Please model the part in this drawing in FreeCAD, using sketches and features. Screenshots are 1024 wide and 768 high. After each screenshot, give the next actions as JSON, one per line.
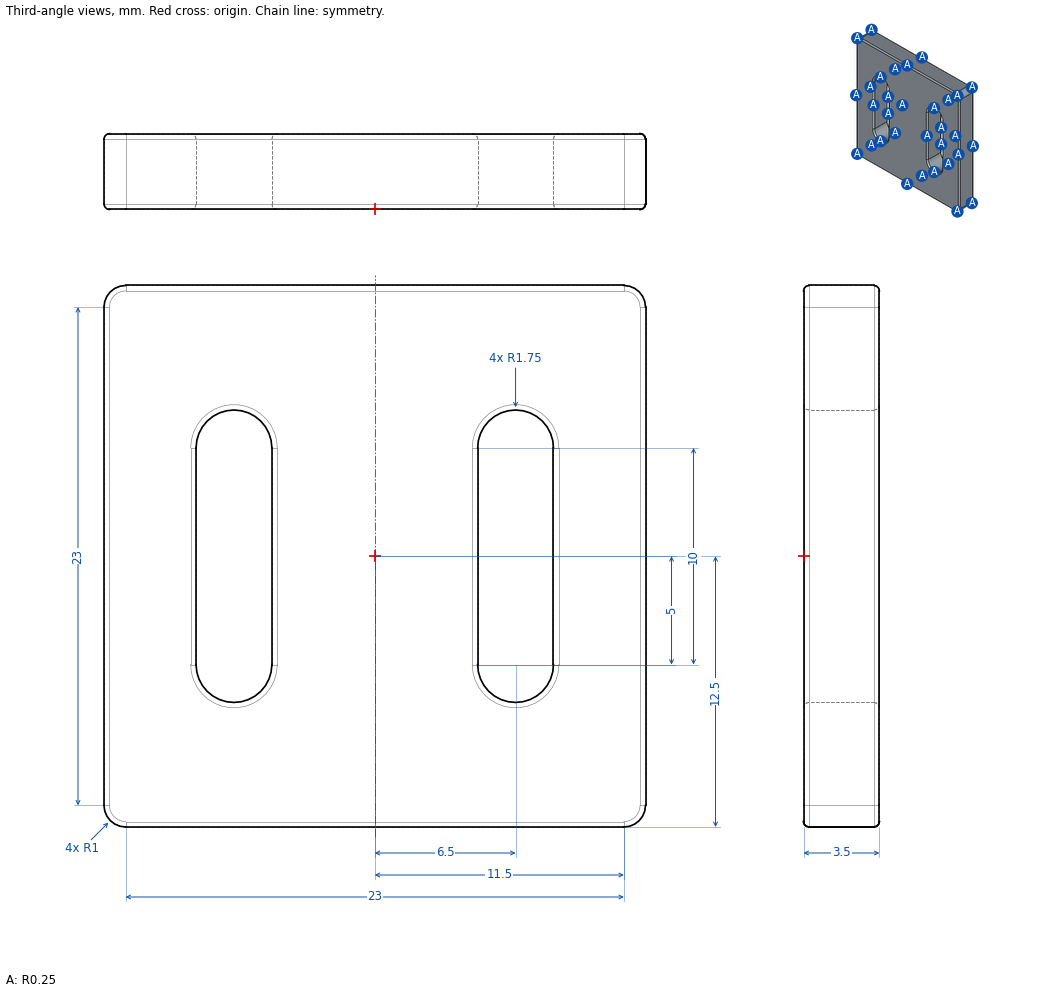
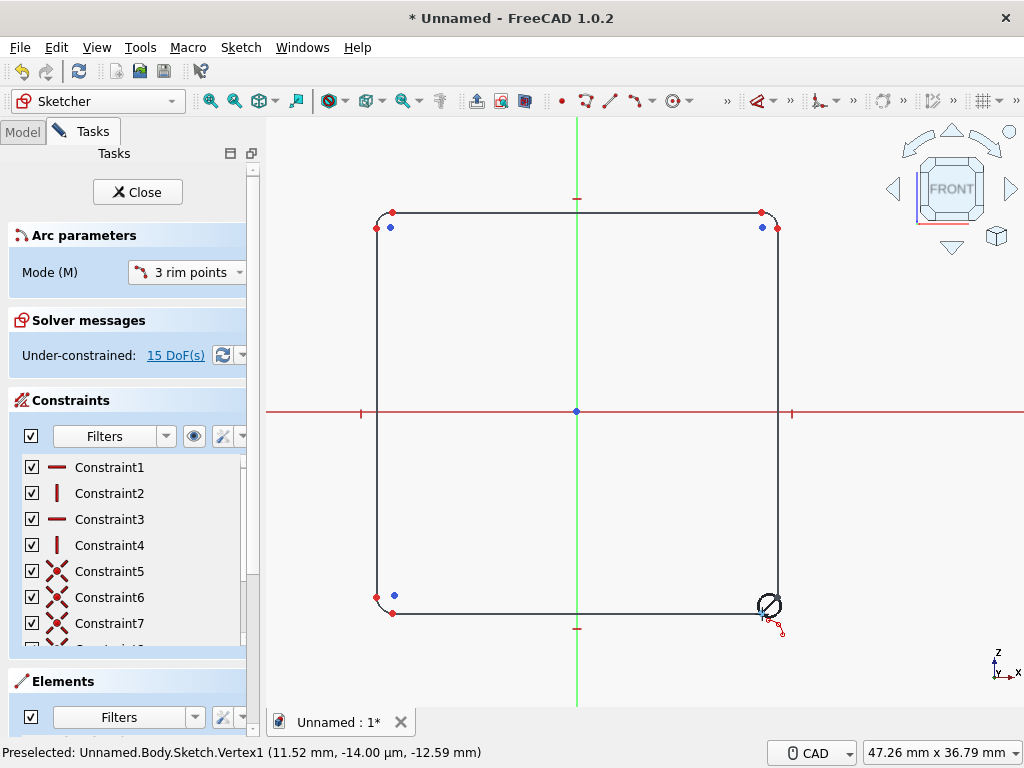
{"action": "scroll", "coordinate": [773, 608], "scroll_direction": "up", "scroll_amount": 7}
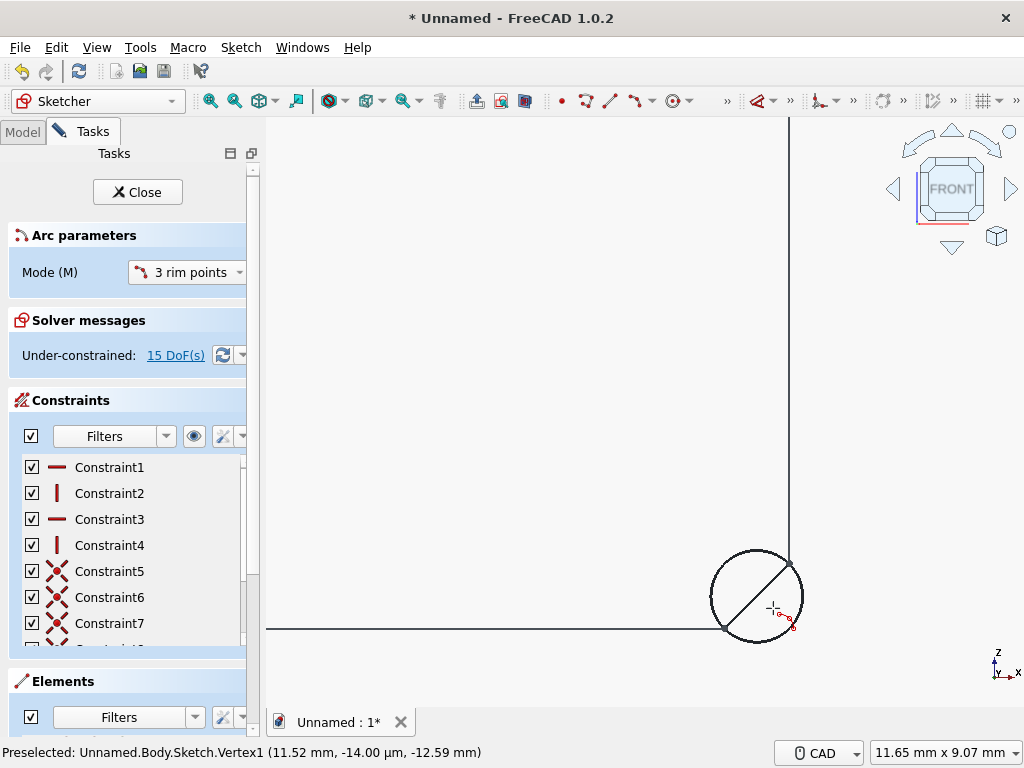
{"action": "left_click", "coordinate": [769, 604]}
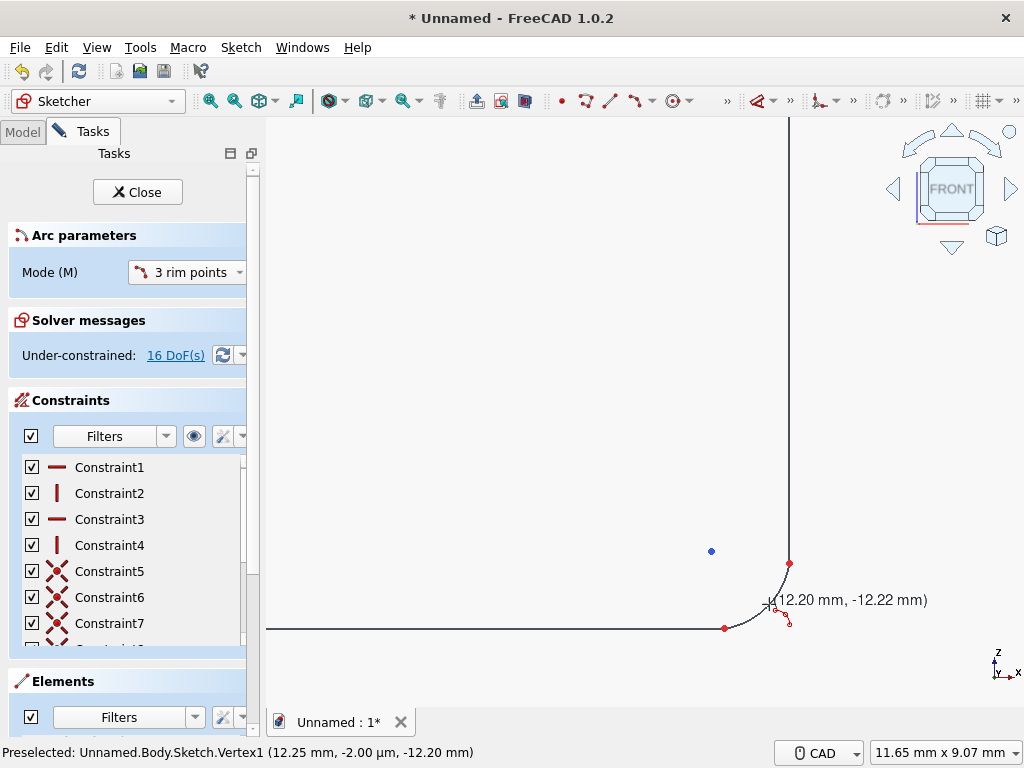
{"action": "key", "text": "g s"}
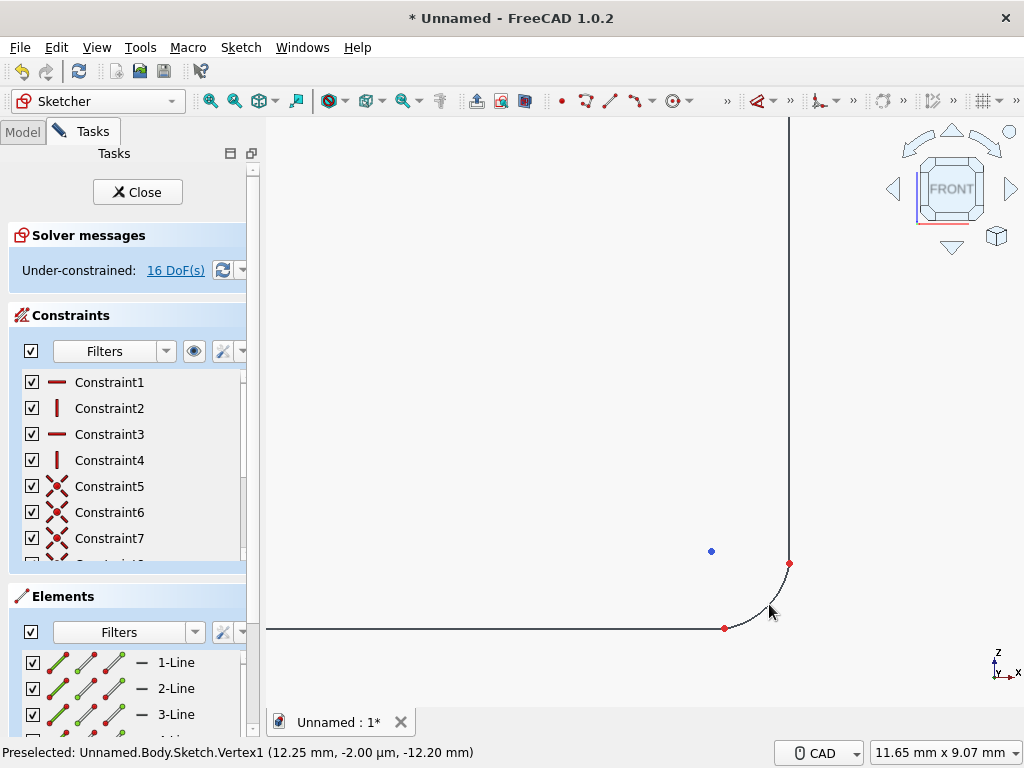
{"action": "scroll", "coordinate": [773, 609], "scroll_direction": "down", "scroll_amount": 7}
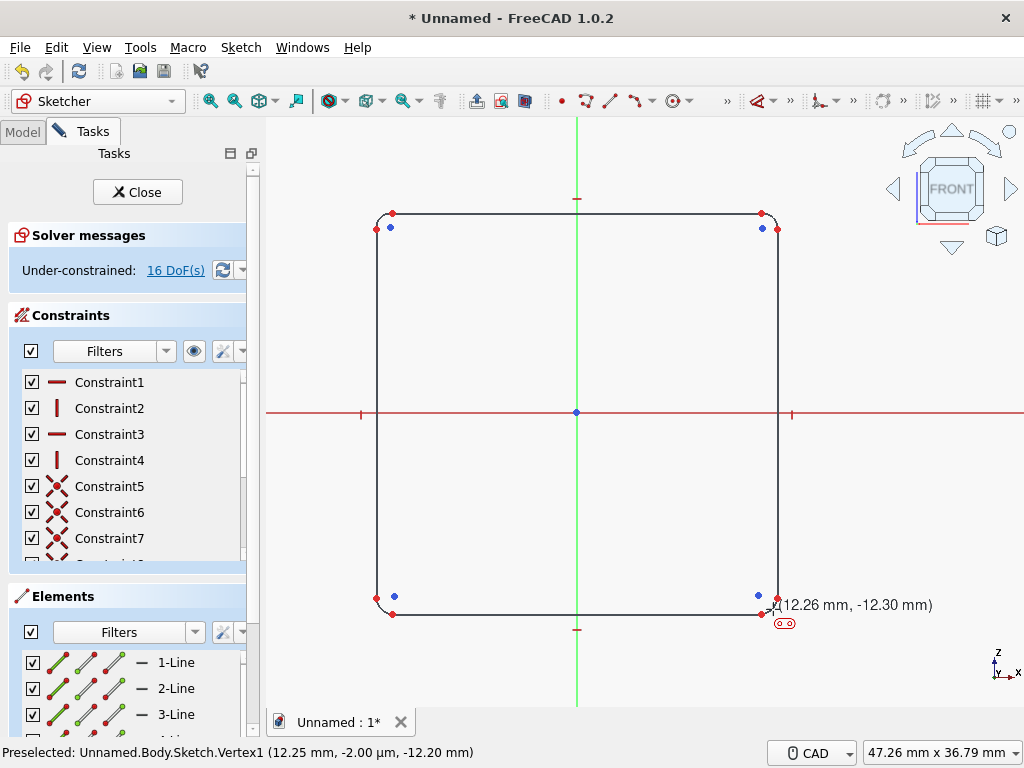
{"action": "left_click", "coordinate": [681, 493]}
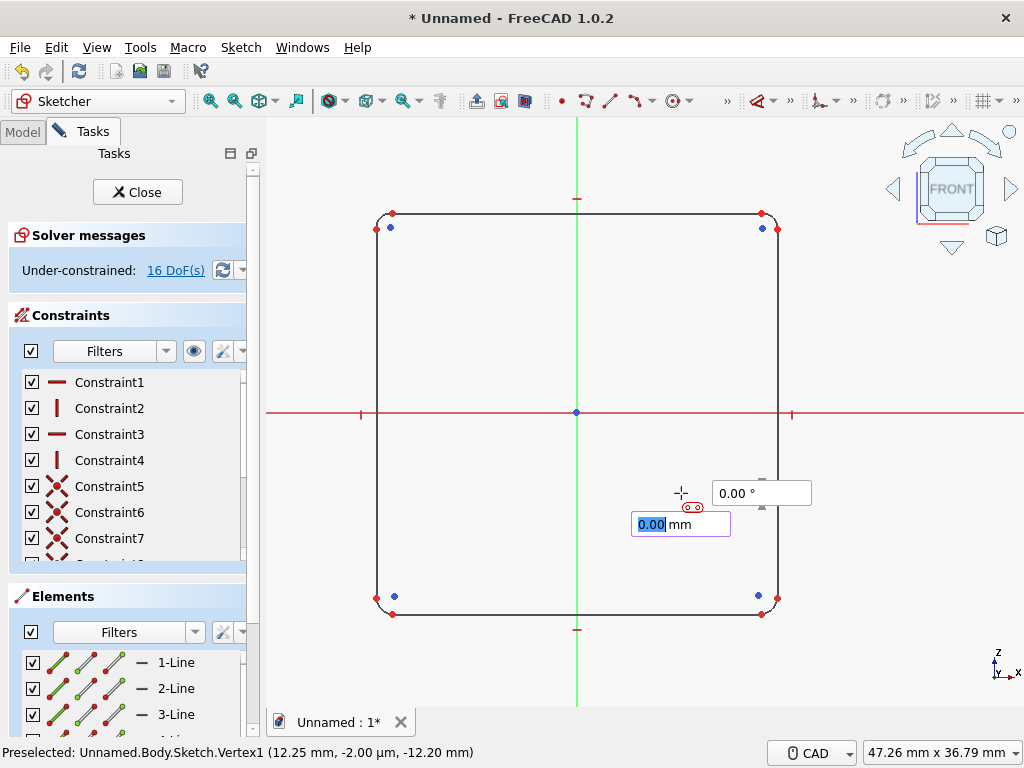
{"action": "left_click", "coordinate": [681, 332]}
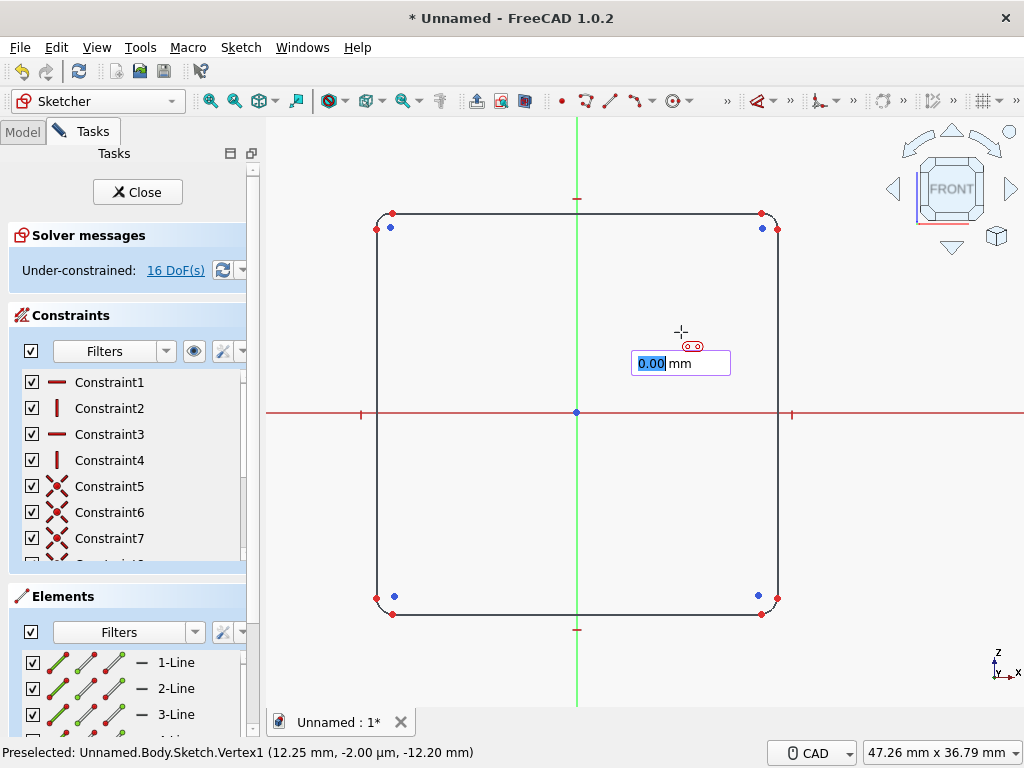
{"action": "left_click", "coordinate": [653, 389]}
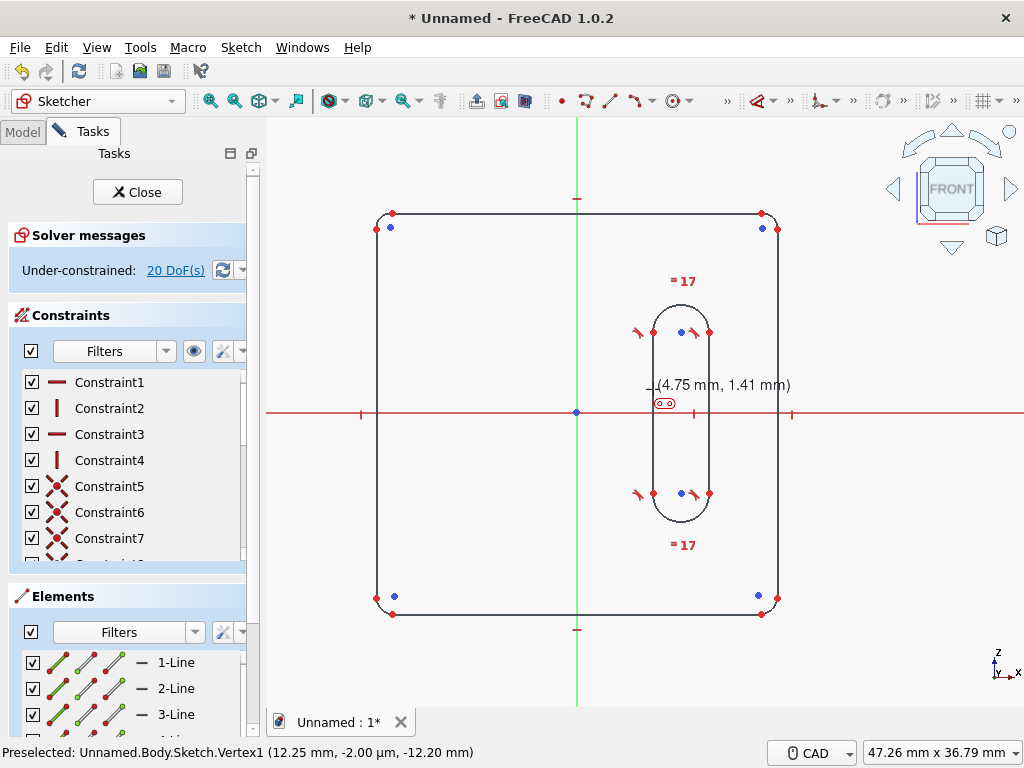
{"action": "left_click", "coordinate": [473, 493]}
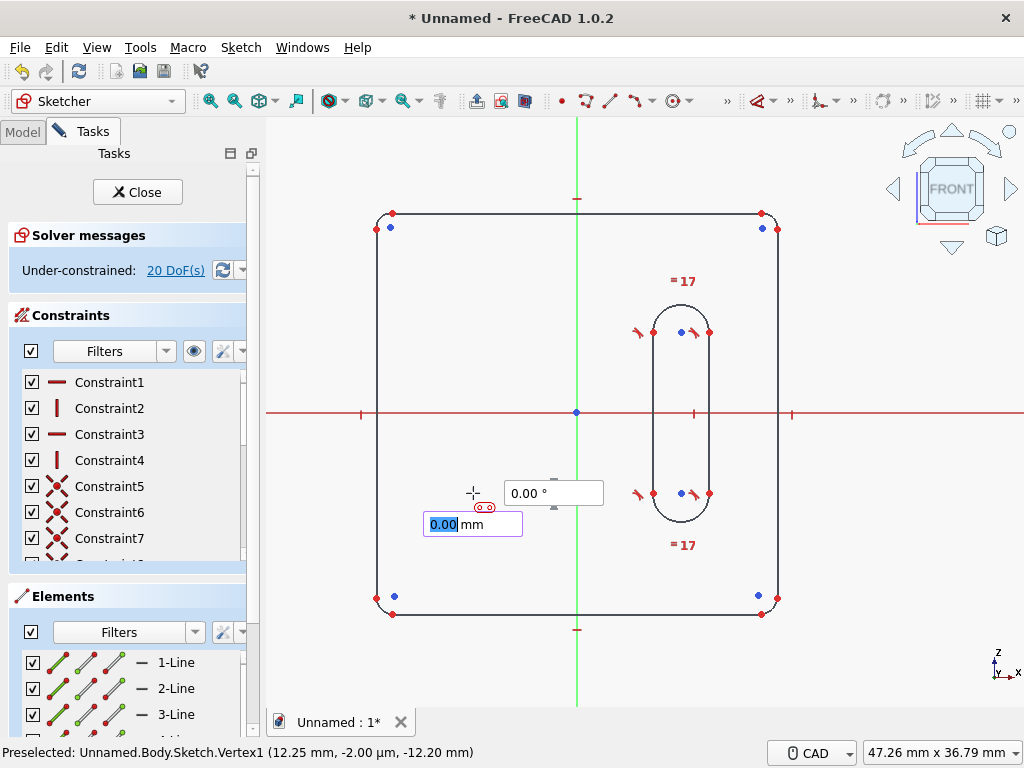
{"action": "left_click", "coordinate": [473, 332]}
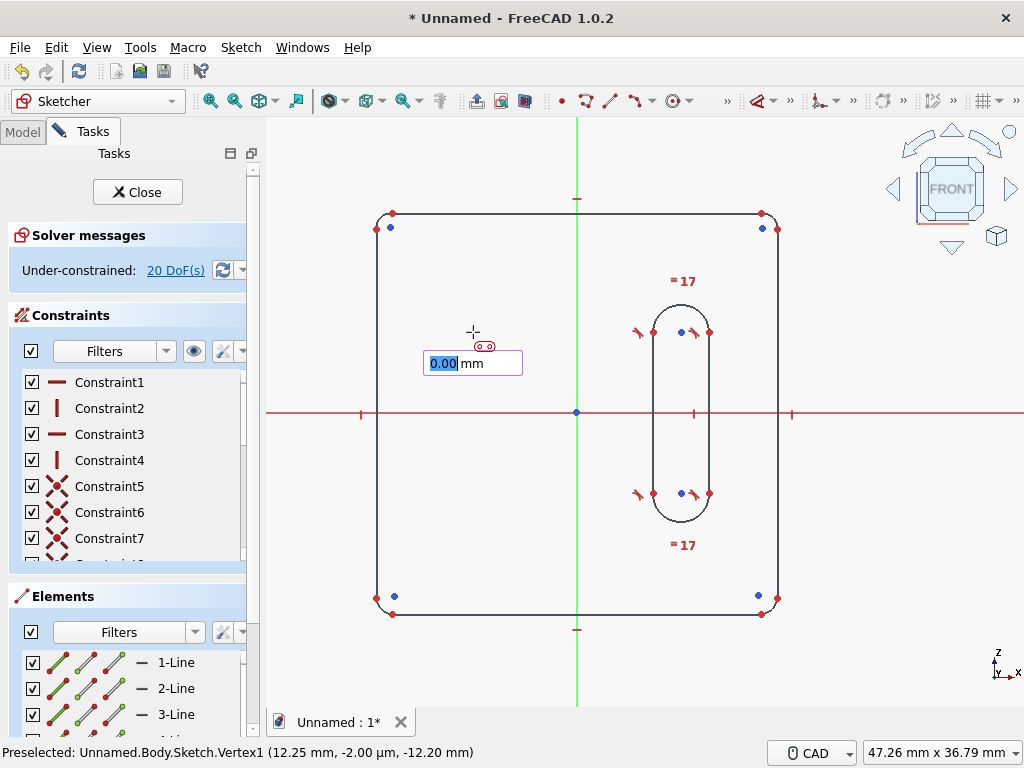
{"action": "left_click", "coordinate": [445, 389]}
{"action": "key", "text": "Escape"}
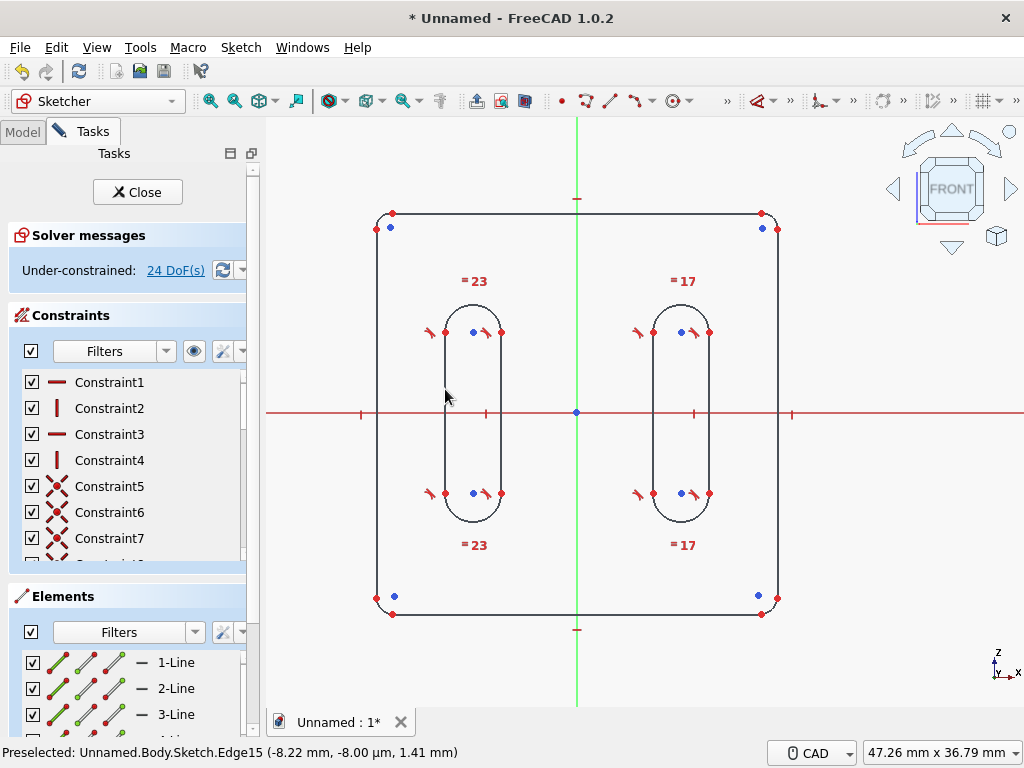
{"action": "left_click", "coordinate": [651, 615]}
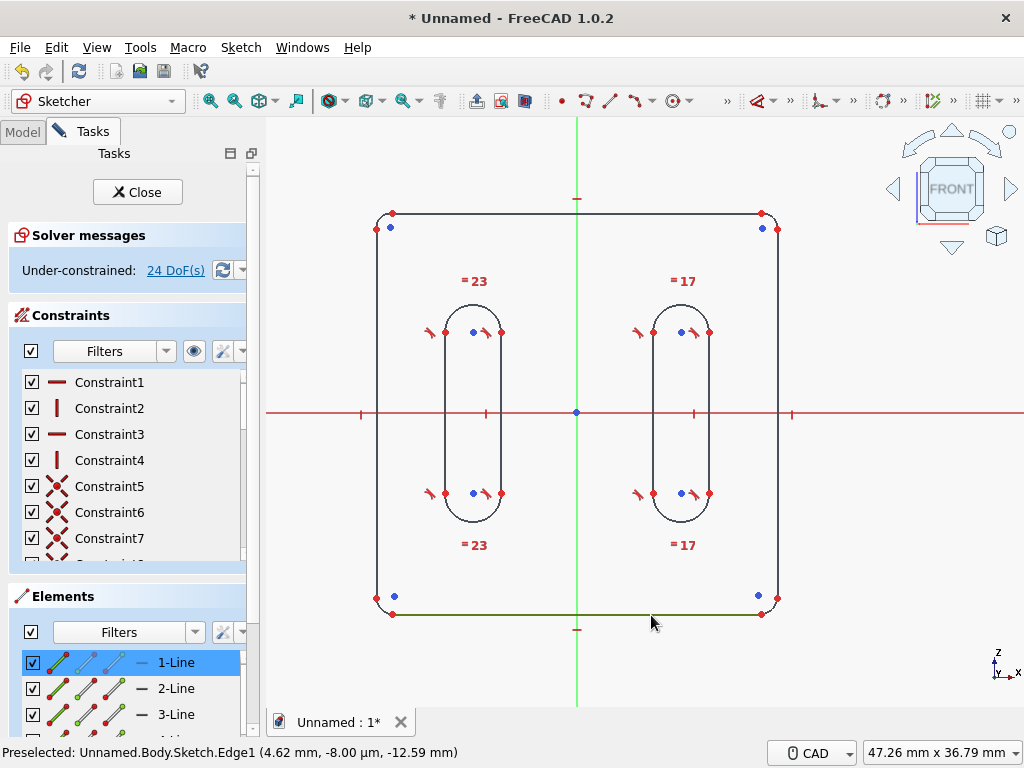
{"action": "left_click", "coordinate": [382, 609]}